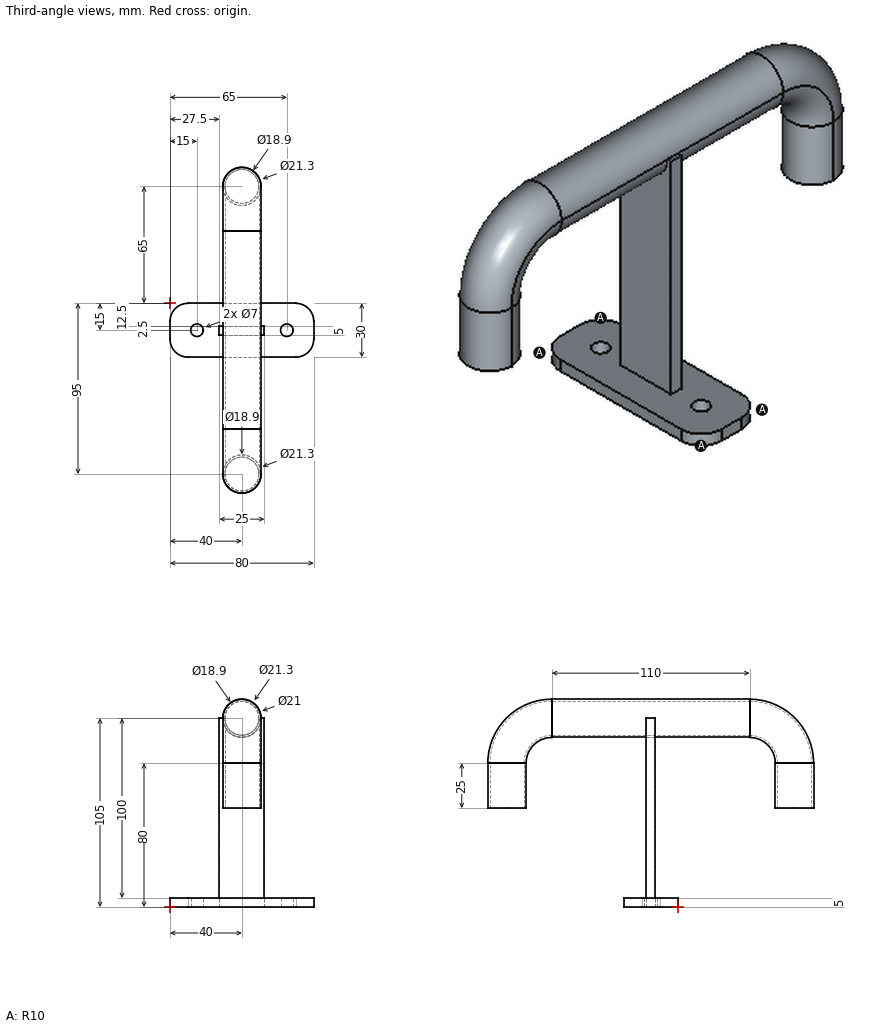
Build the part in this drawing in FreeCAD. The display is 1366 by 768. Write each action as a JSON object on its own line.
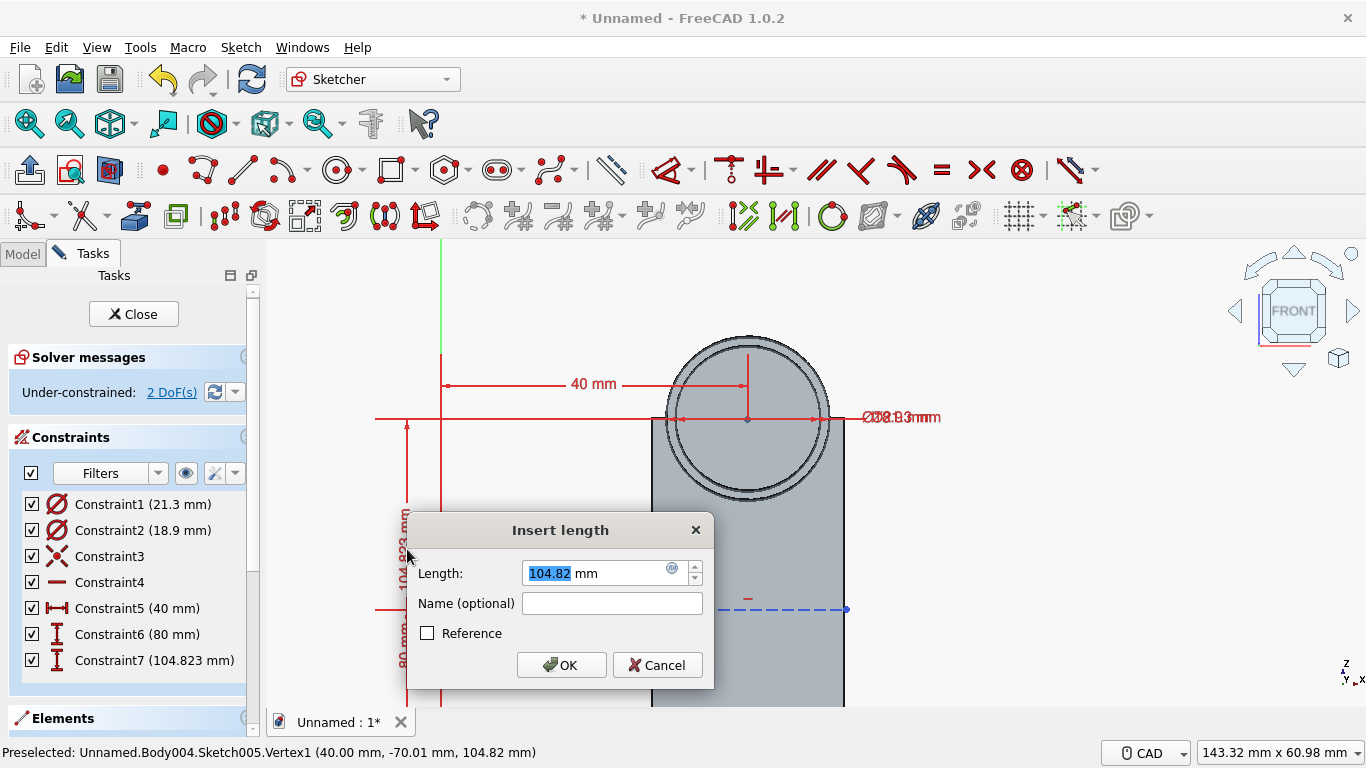
{"action": "type", "text": "105"}
{"action": "key", "text": "Return"}
{"action": "key", "text": "Escape"}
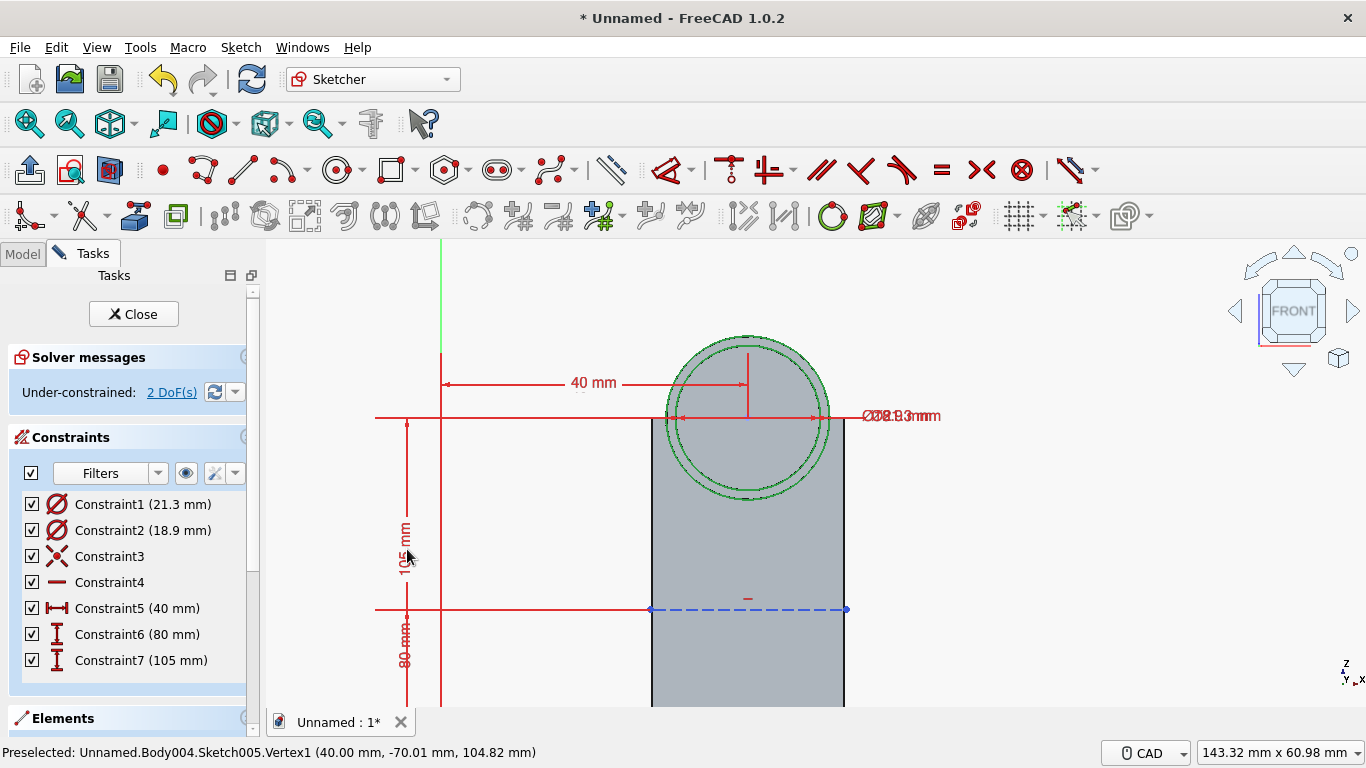
{"action": "left_click", "coordinate": [134, 314]}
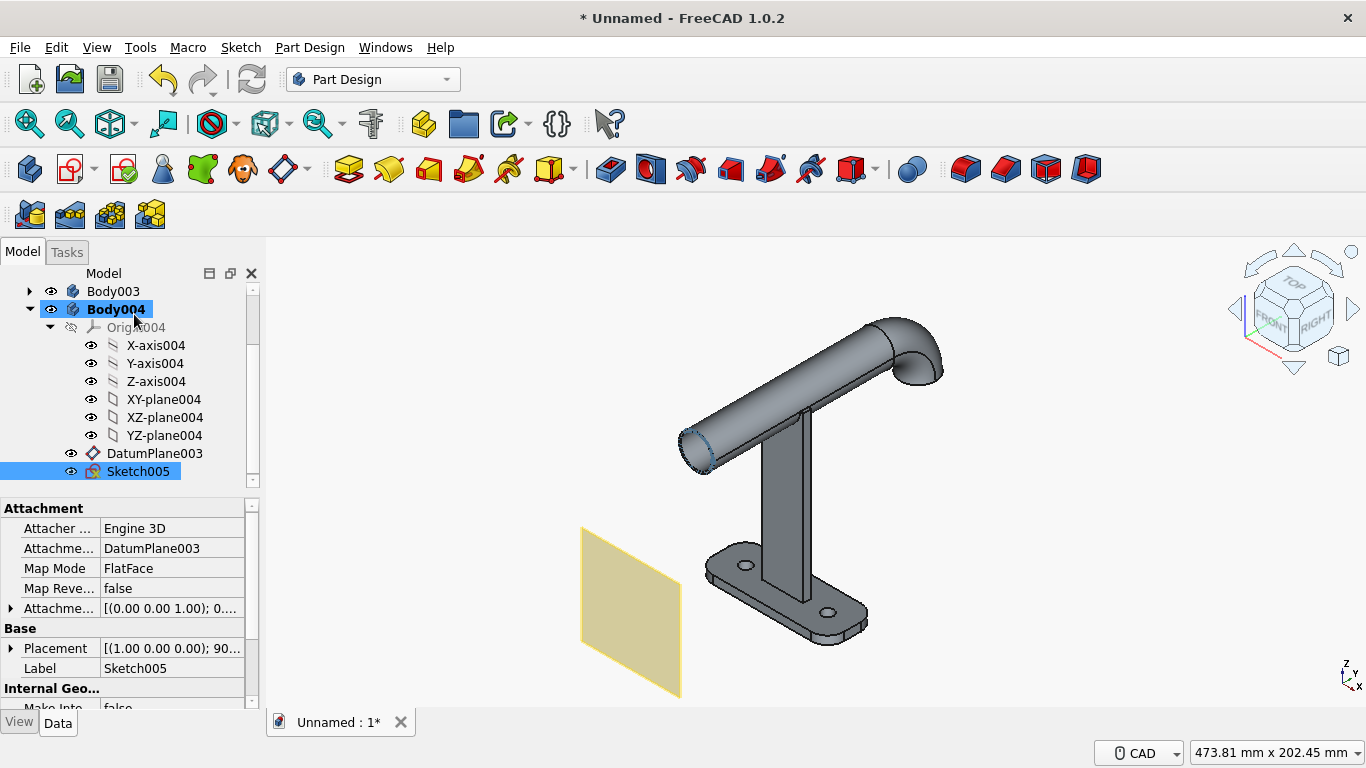
{"action": "left_click", "coordinate": [390, 170]}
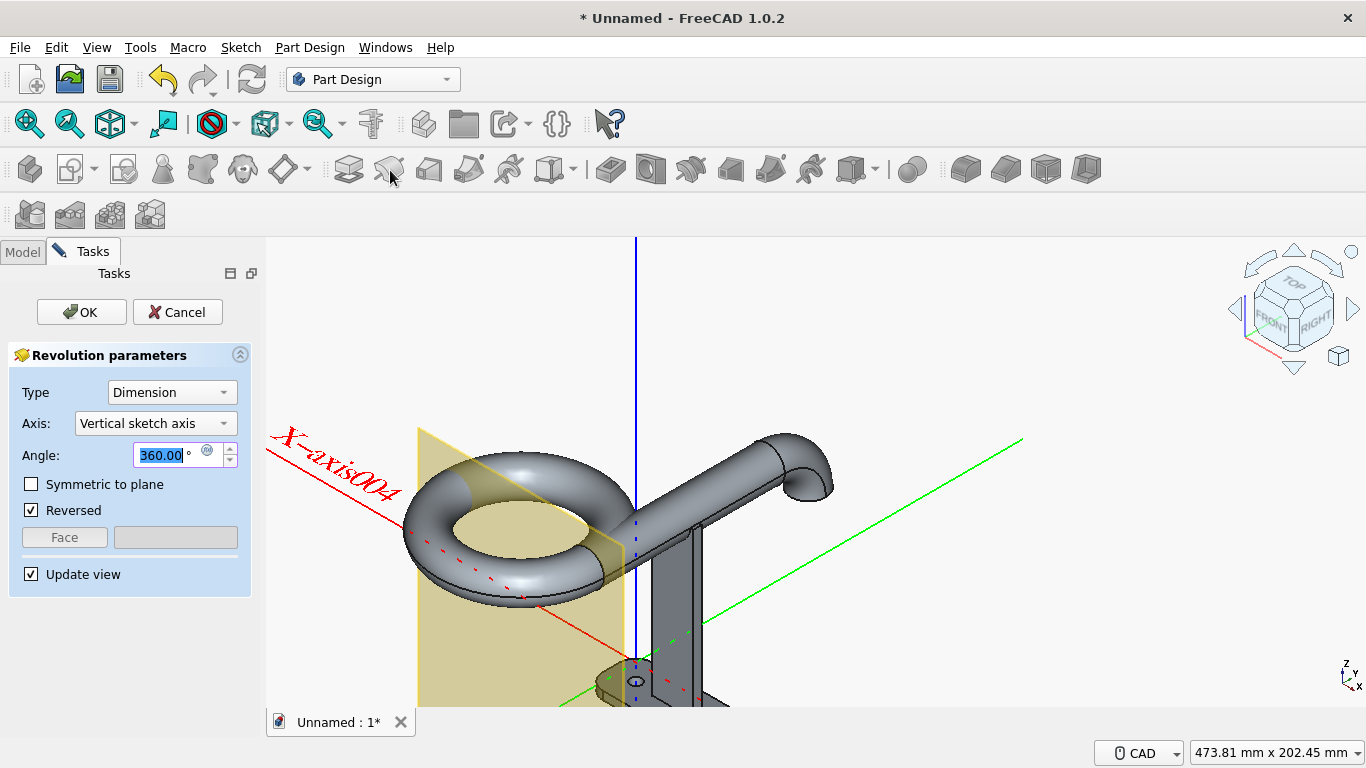
{"action": "left_click", "coordinate": [156, 424]}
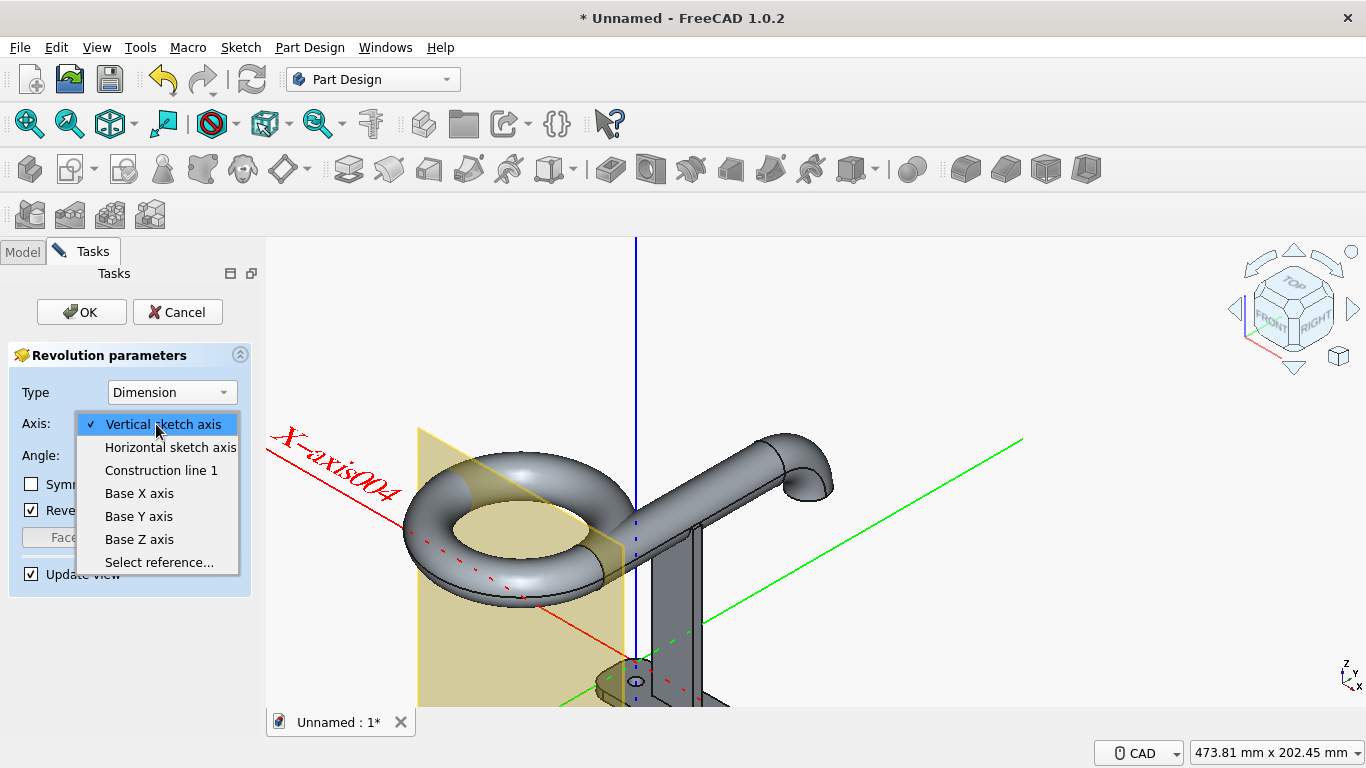
{"action": "left_click", "coordinate": [156, 470]}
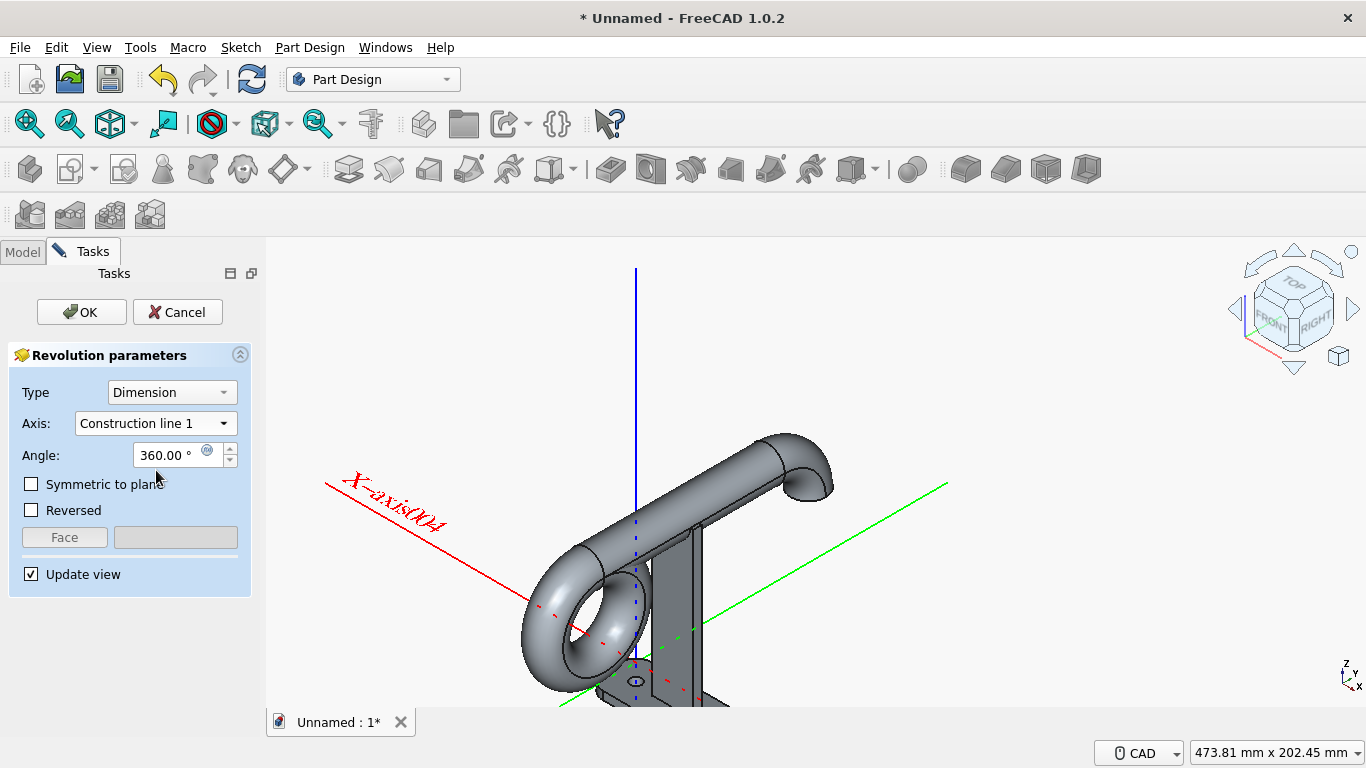
{"action": "triple_click", "coordinate": [178, 455]}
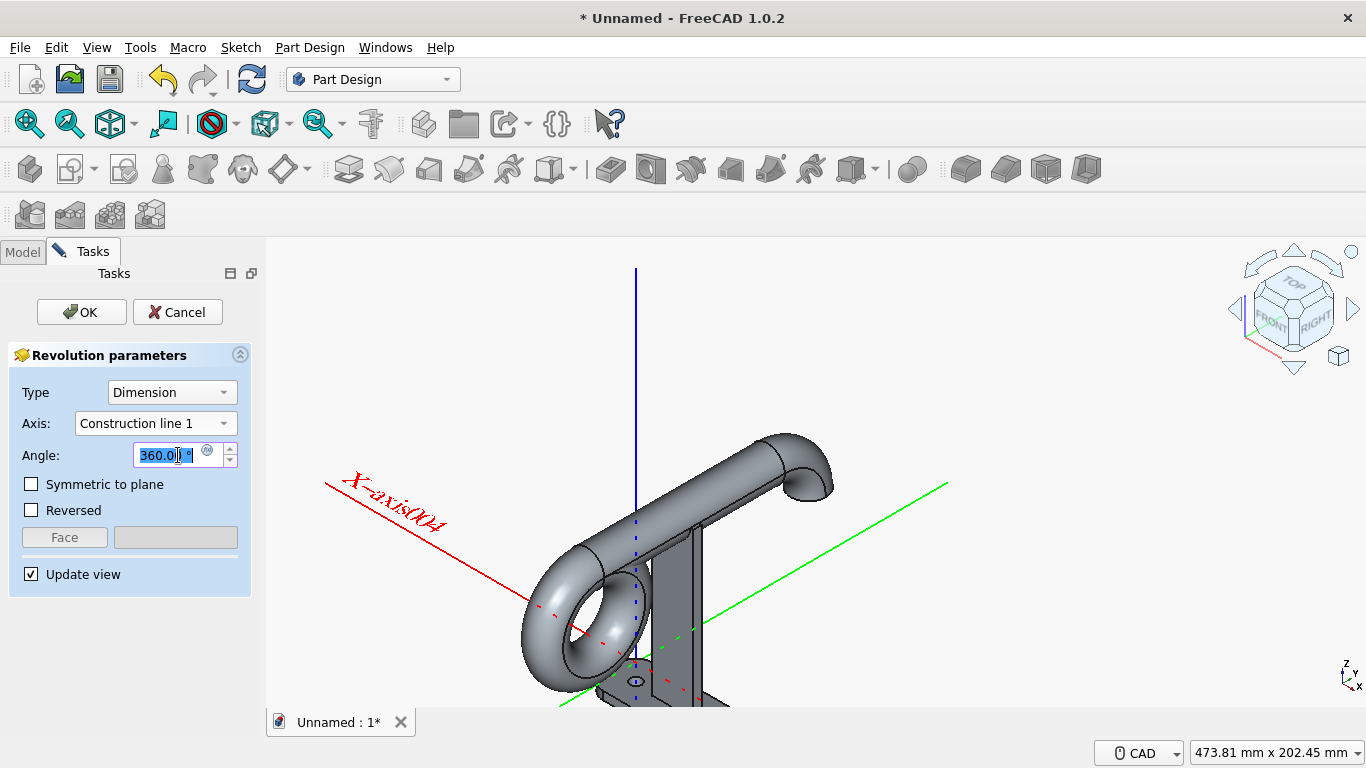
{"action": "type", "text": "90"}
{"action": "key", "text": "Tab"}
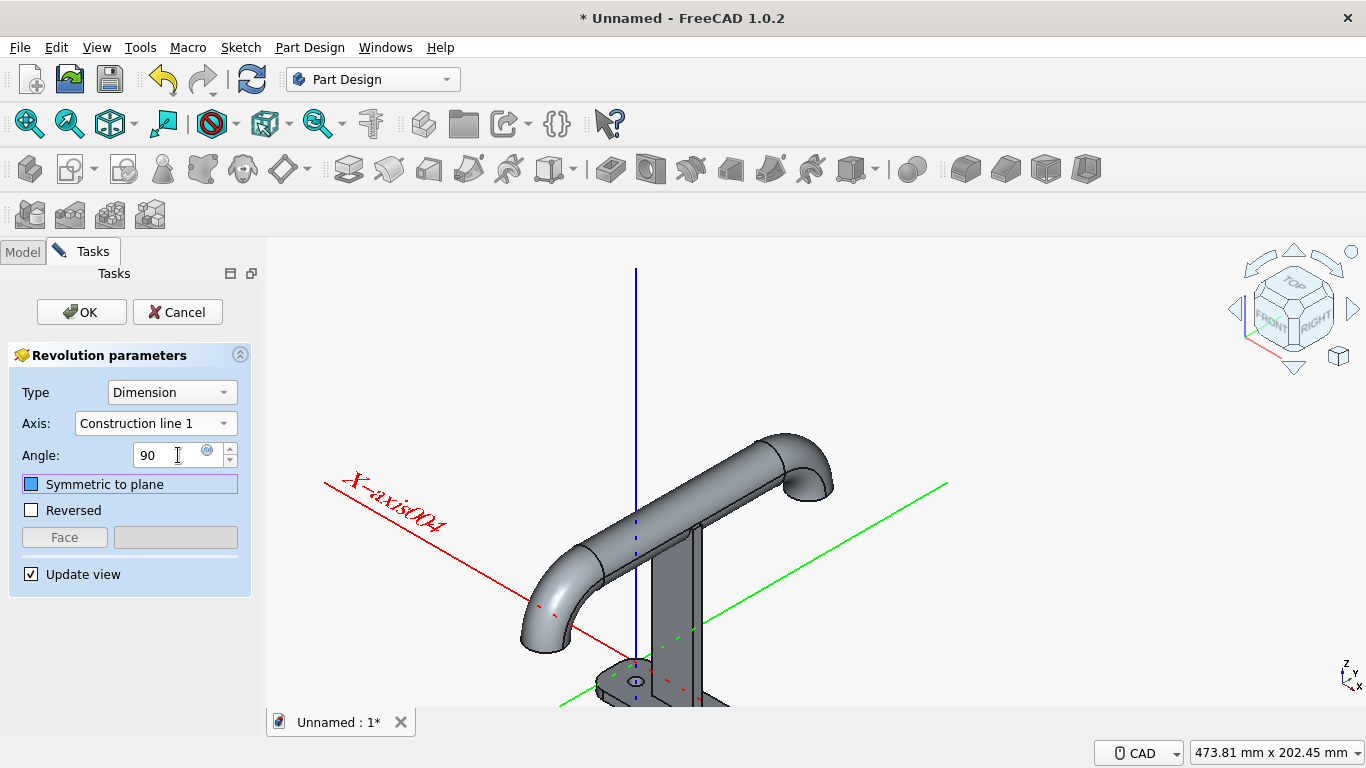
{"action": "left_click", "coordinate": [82, 312]}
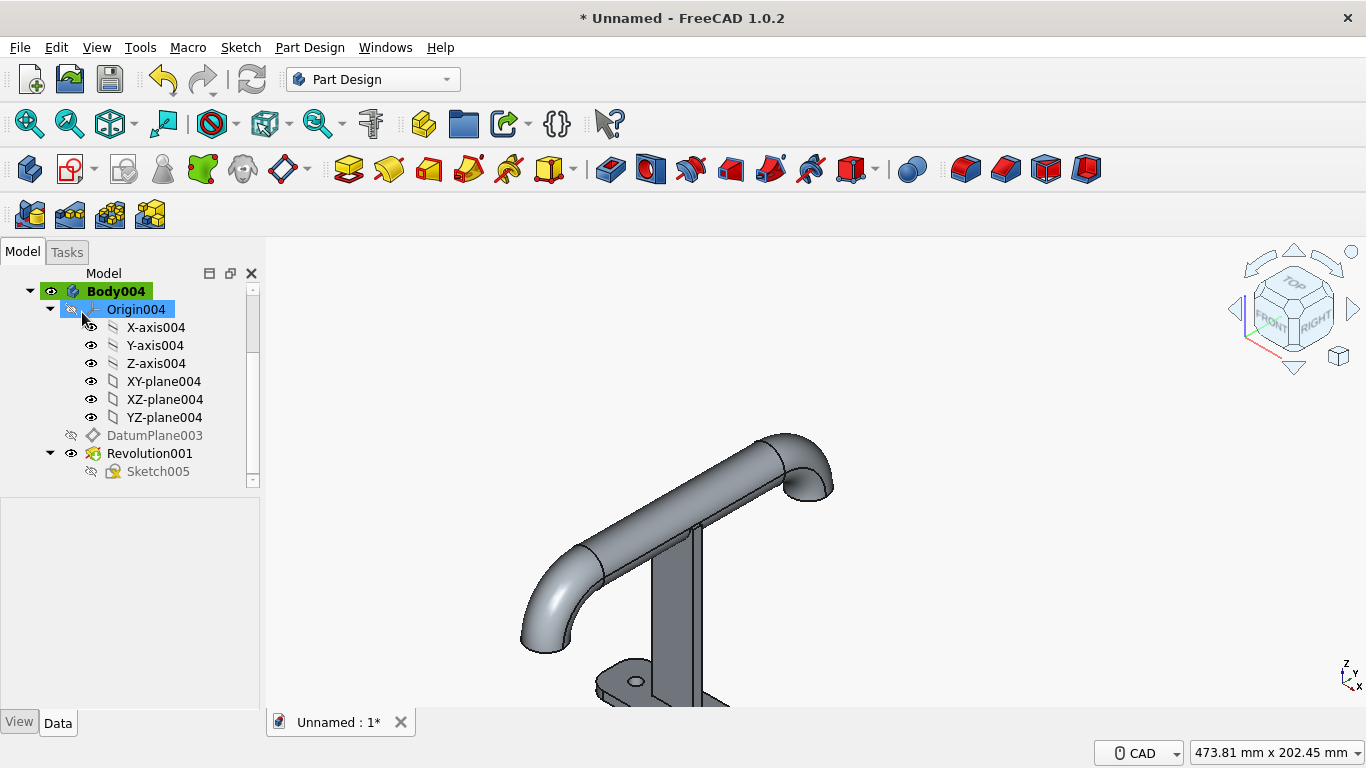
{"action": "left_click", "coordinate": [30, 124]}